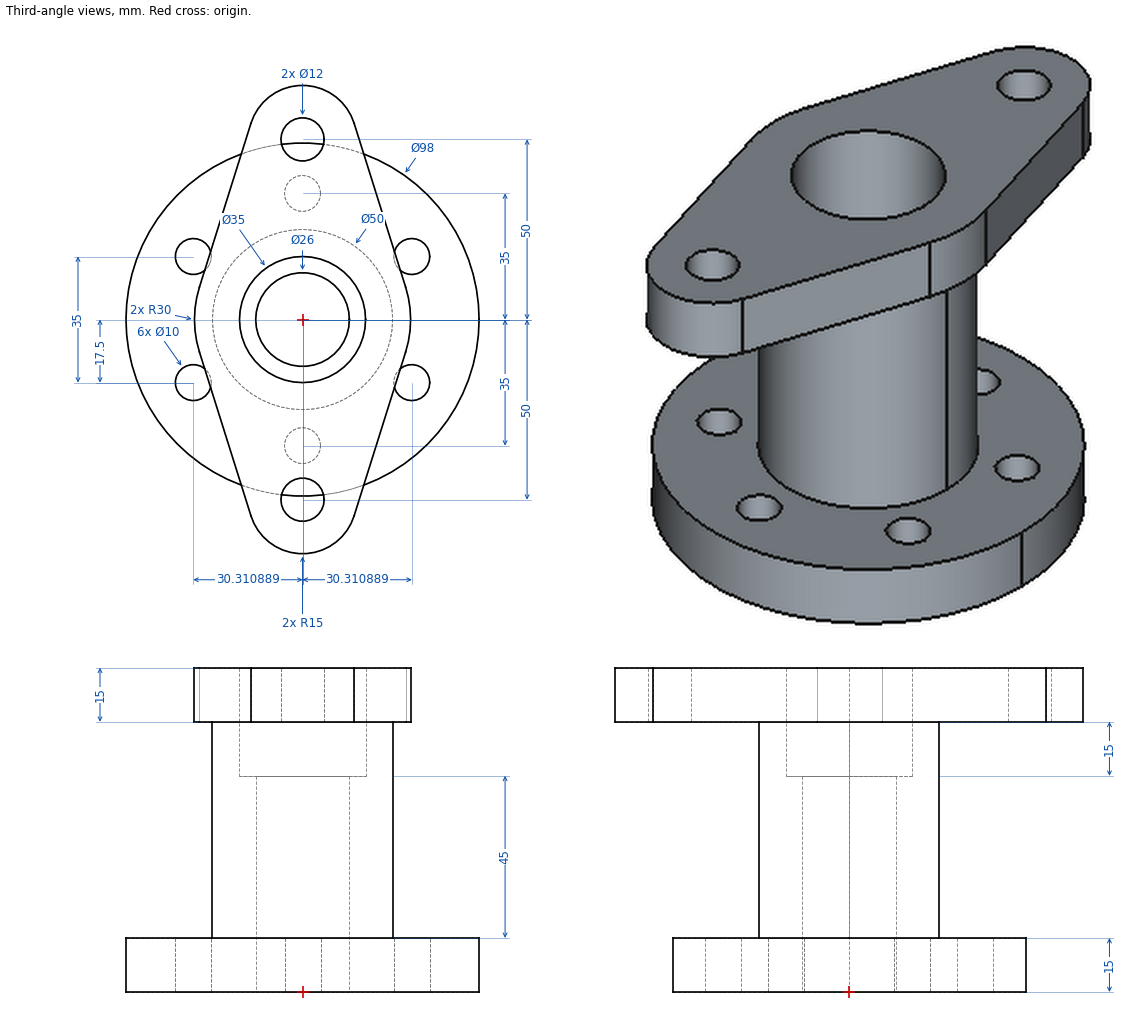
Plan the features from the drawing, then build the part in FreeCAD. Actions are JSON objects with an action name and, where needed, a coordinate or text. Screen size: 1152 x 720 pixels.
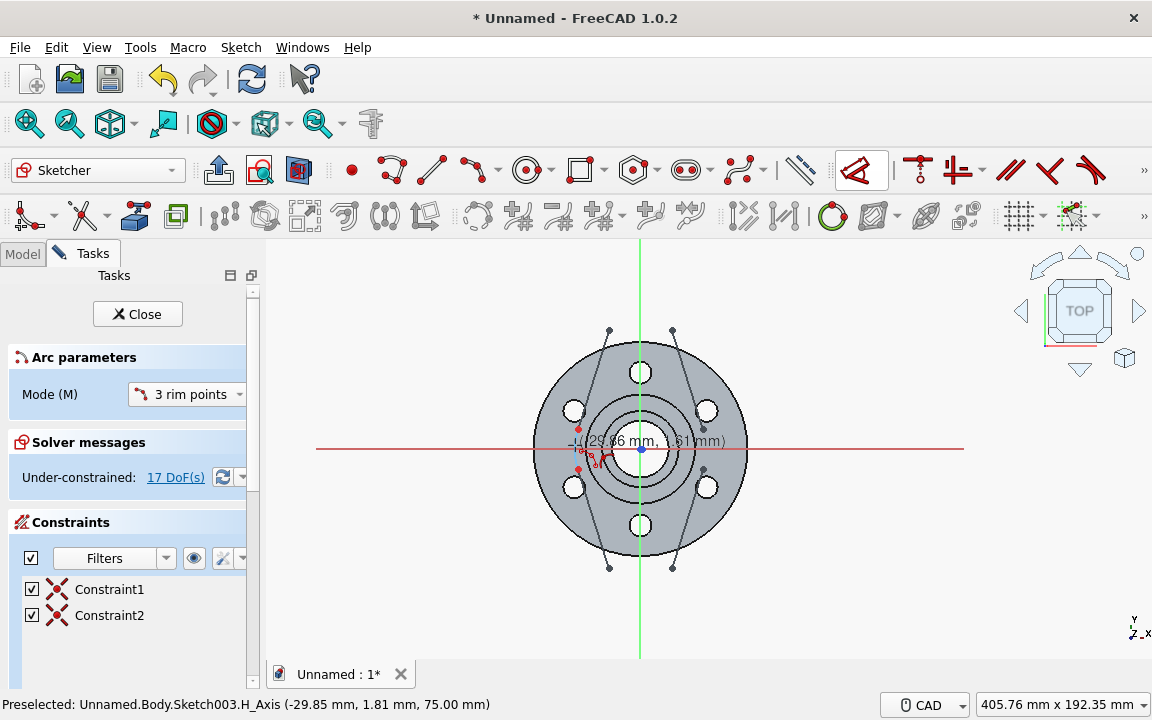
{"action": "left_click", "coordinate": [609, 569]}
{"action": "left_click", "coordinate": [672, 569]}
{"action": "left_click", "coordinate": [625, 587]}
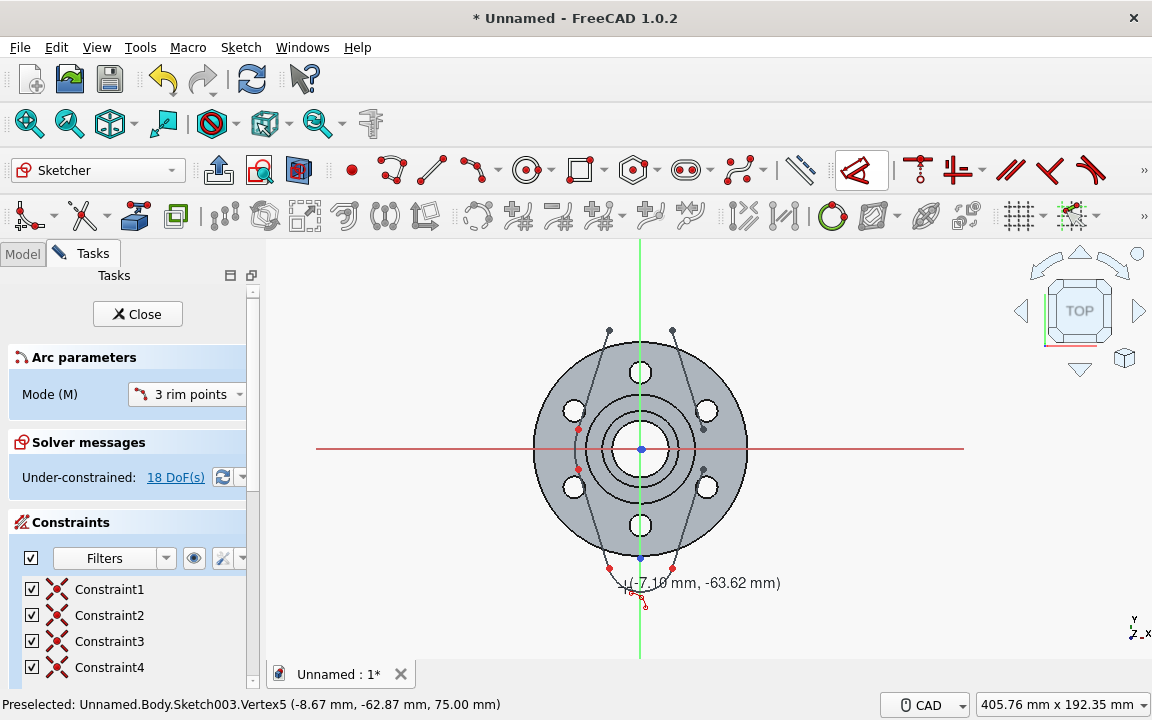
{"action": "left_click", "coordinate": [703, 470]}
{"action": "left_click", "coordinate": [703, 430]}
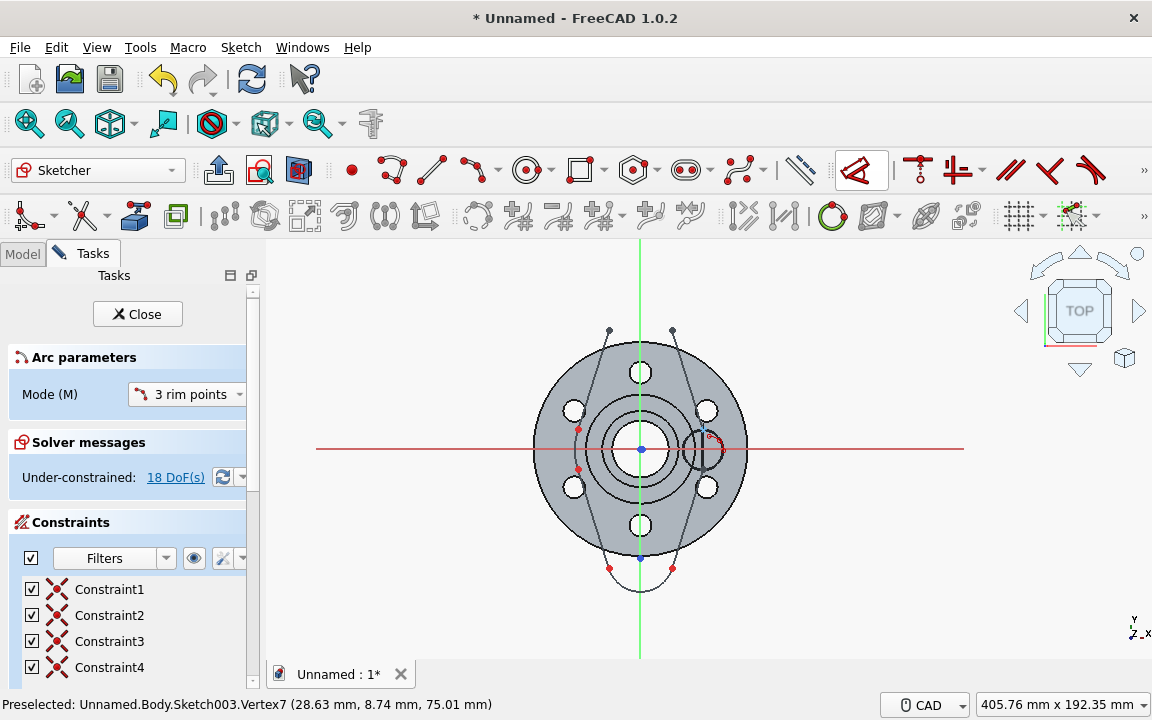
{"action": "scroll", "coordinate": [706, 453], "scroll_direction": "up", "scroll_amount": 9}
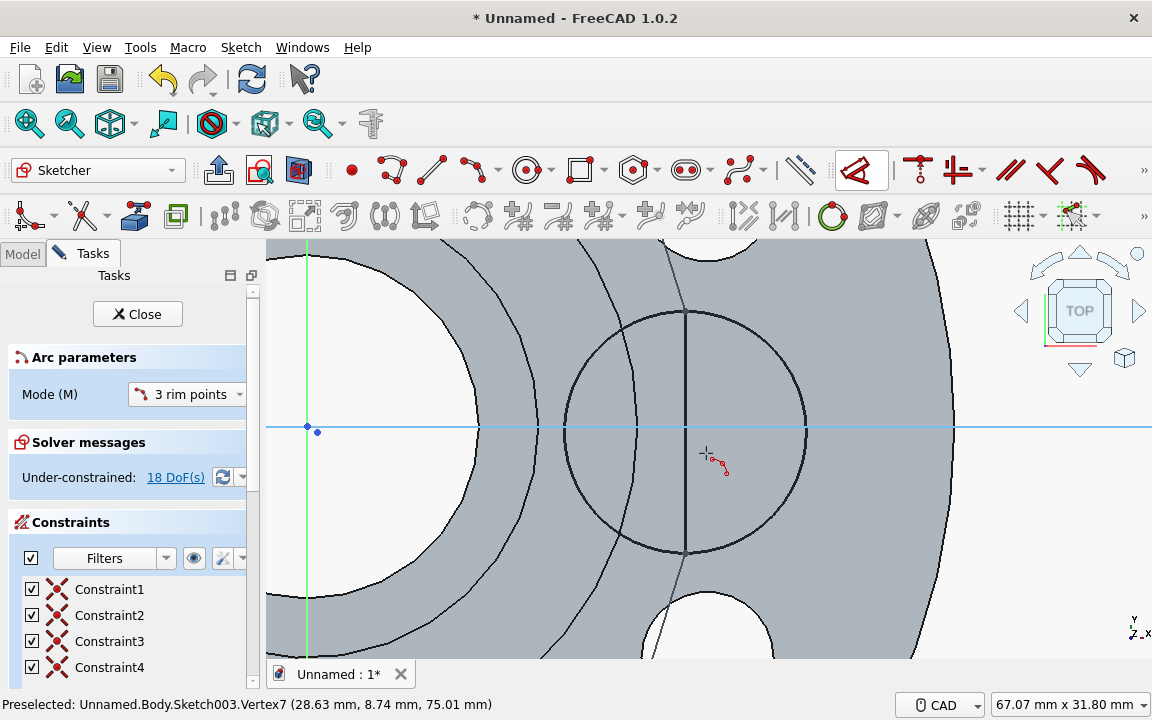
{"action": "left_click", "coordinate": [703, 451]}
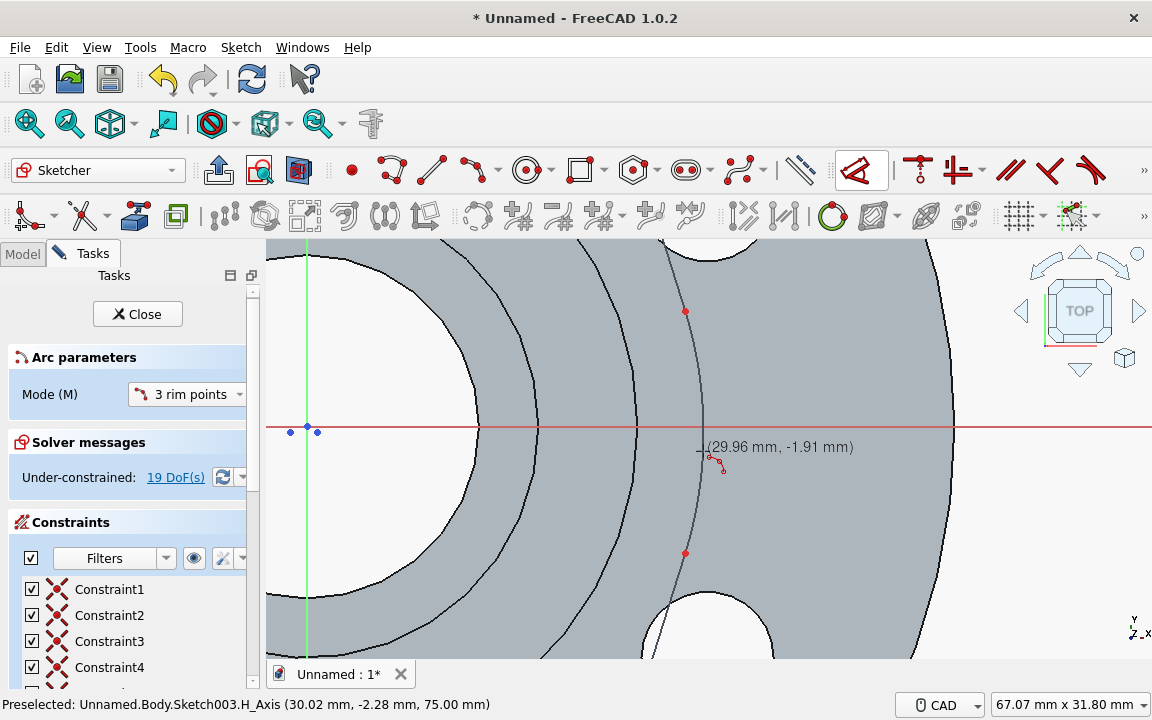
{"action": "scroll", "coordinate": [707, 453], "scroll_direction": "down", "scroll_amount": 9}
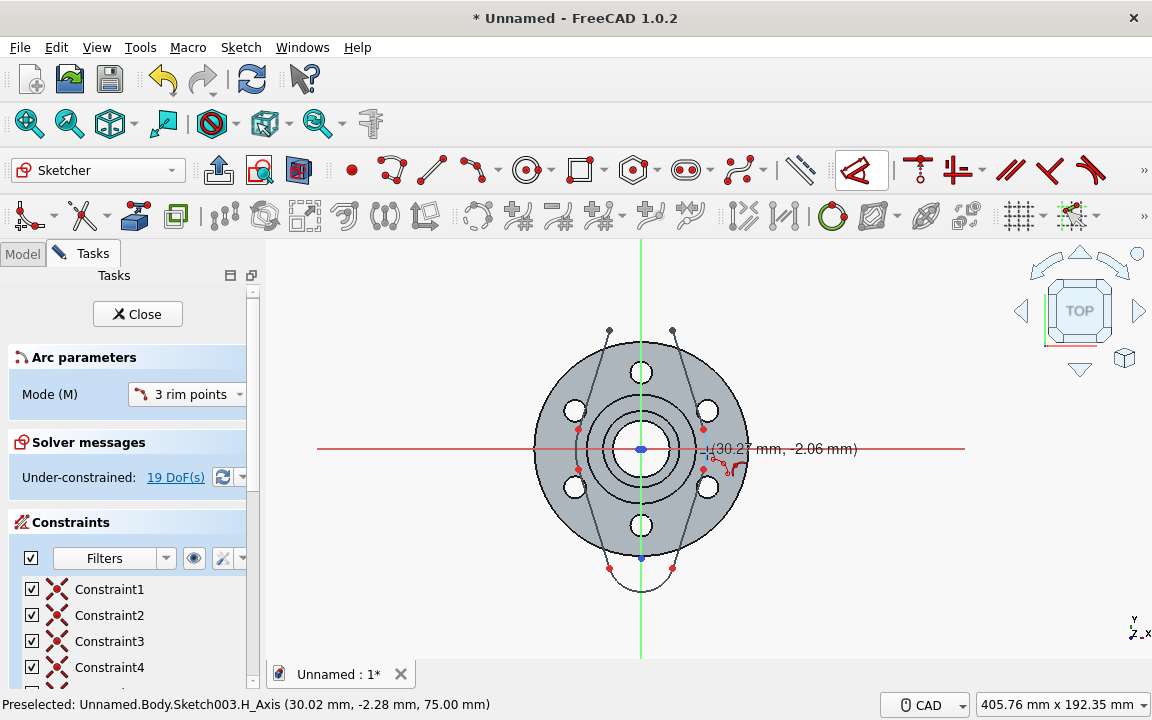
{"action": "left_click", "coordinate": [673, 331]}
{"action": "left_click", "coordinate": [610, 331]}
{"action": "left_click", "coordinate": [657, 311]}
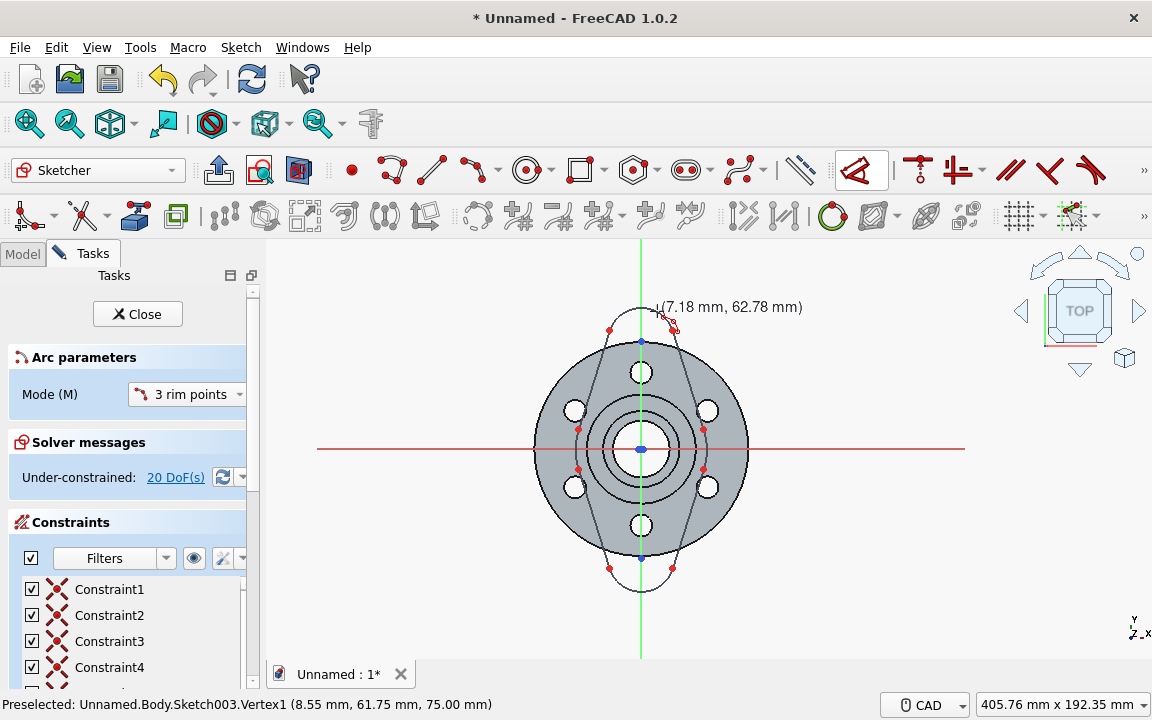
{"action": "key", "text": "g c"}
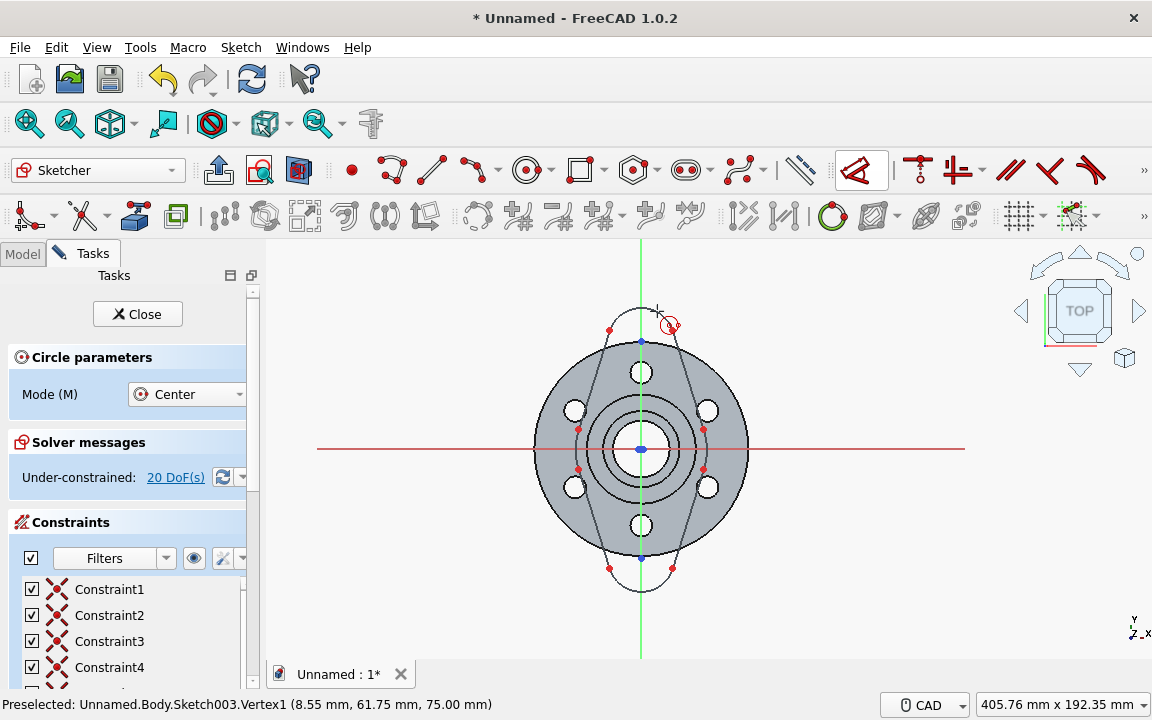
{"action": "scroll", "coordinate": [641, 340], "scroll_direction": "up", "scroll_amount": 3}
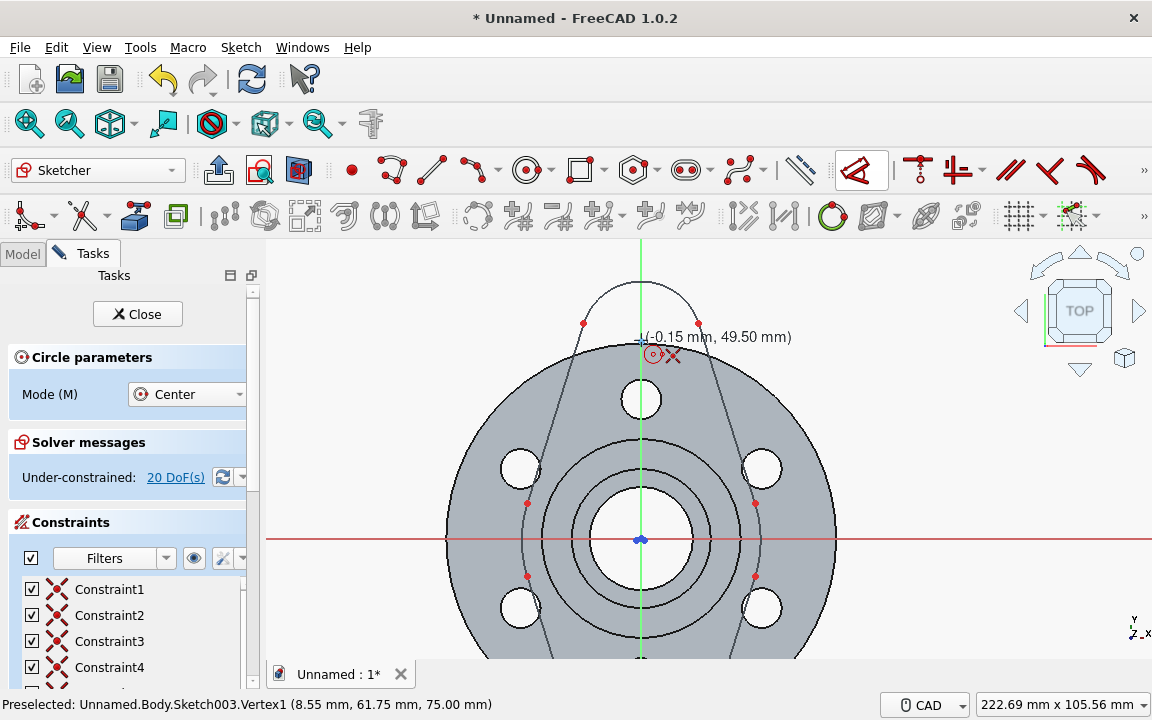
{"action": "left_click", "coordinate": [641, 340]}
{"action": "left_click", "coordinate": [658, 323]}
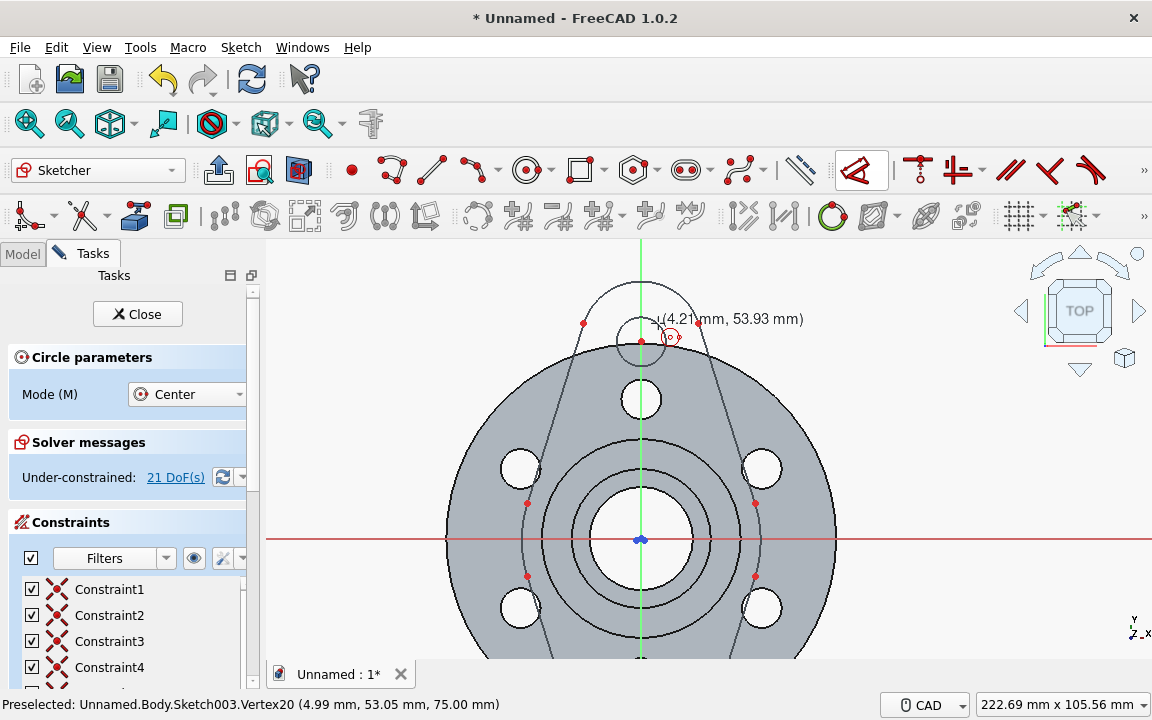
{"action": "scroll", "coordinate": [640, 340], "scroll_direction": "down", "scroll_amount": 3}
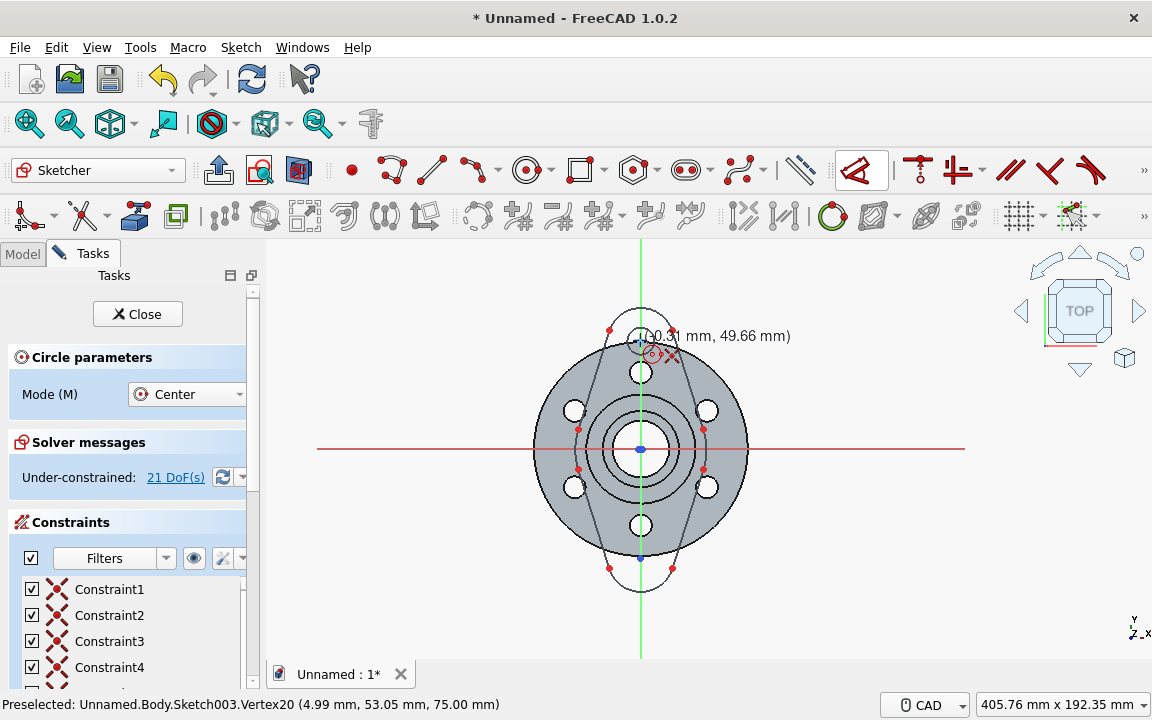
{"action": "scroll", "coordinate": [641, 558], "scroll_direction": "up", "scroll_amount": 3}